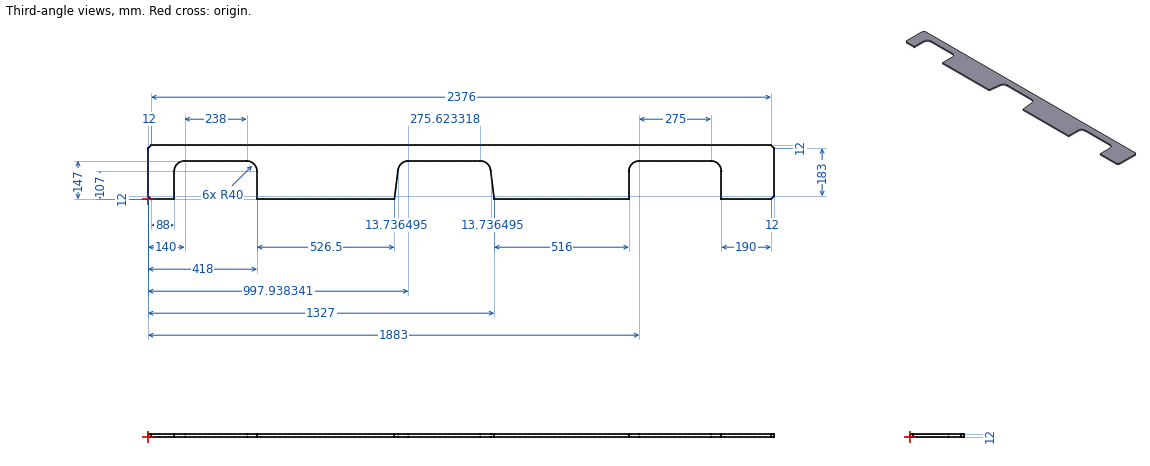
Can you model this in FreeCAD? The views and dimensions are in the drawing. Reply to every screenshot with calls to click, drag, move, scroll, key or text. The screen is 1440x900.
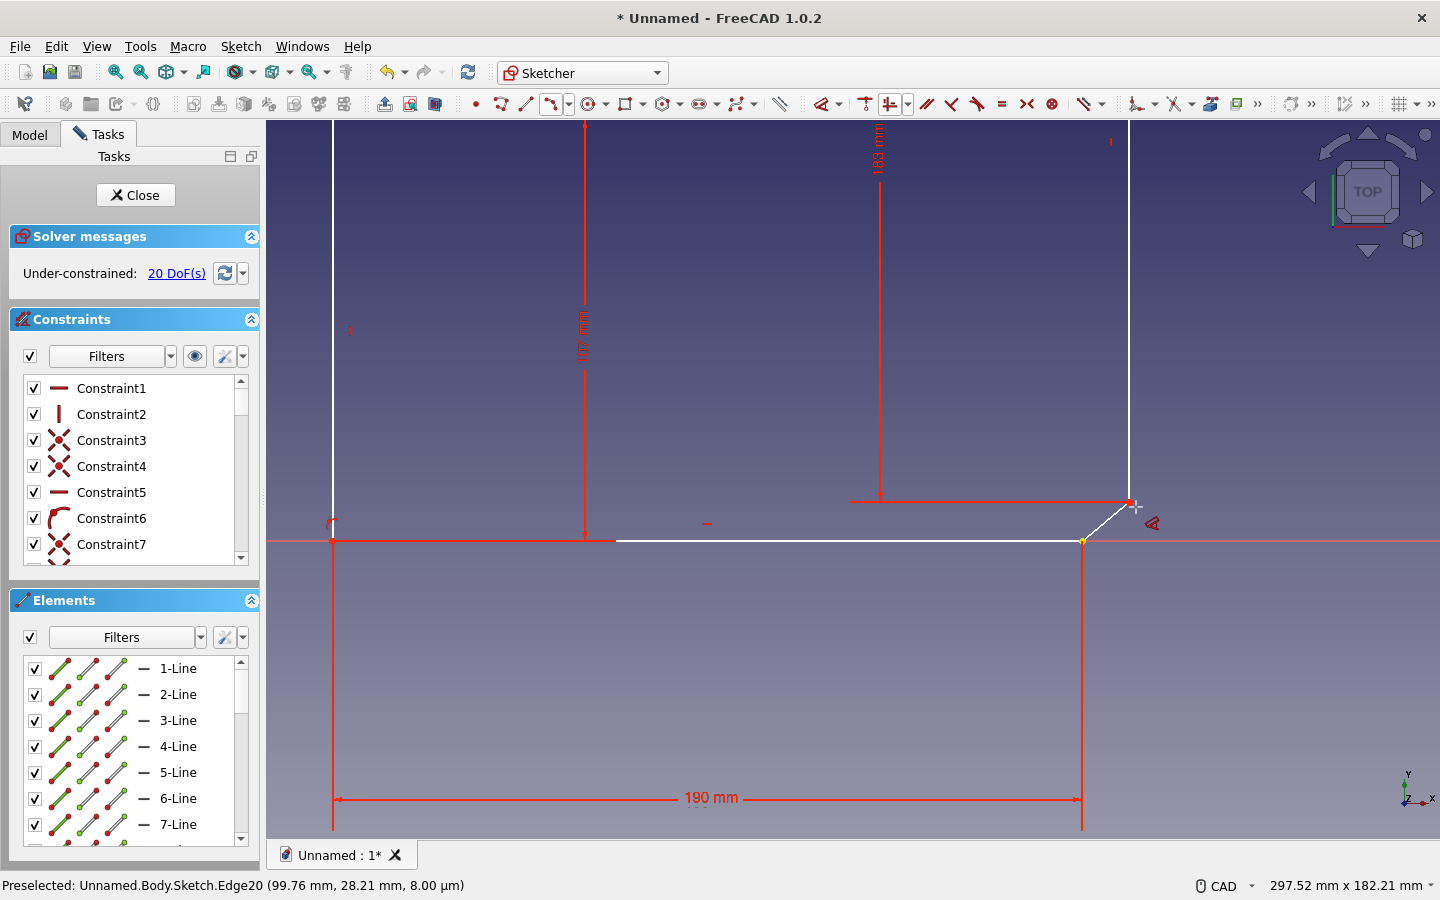
click(1129, 502)
click(1163, 522)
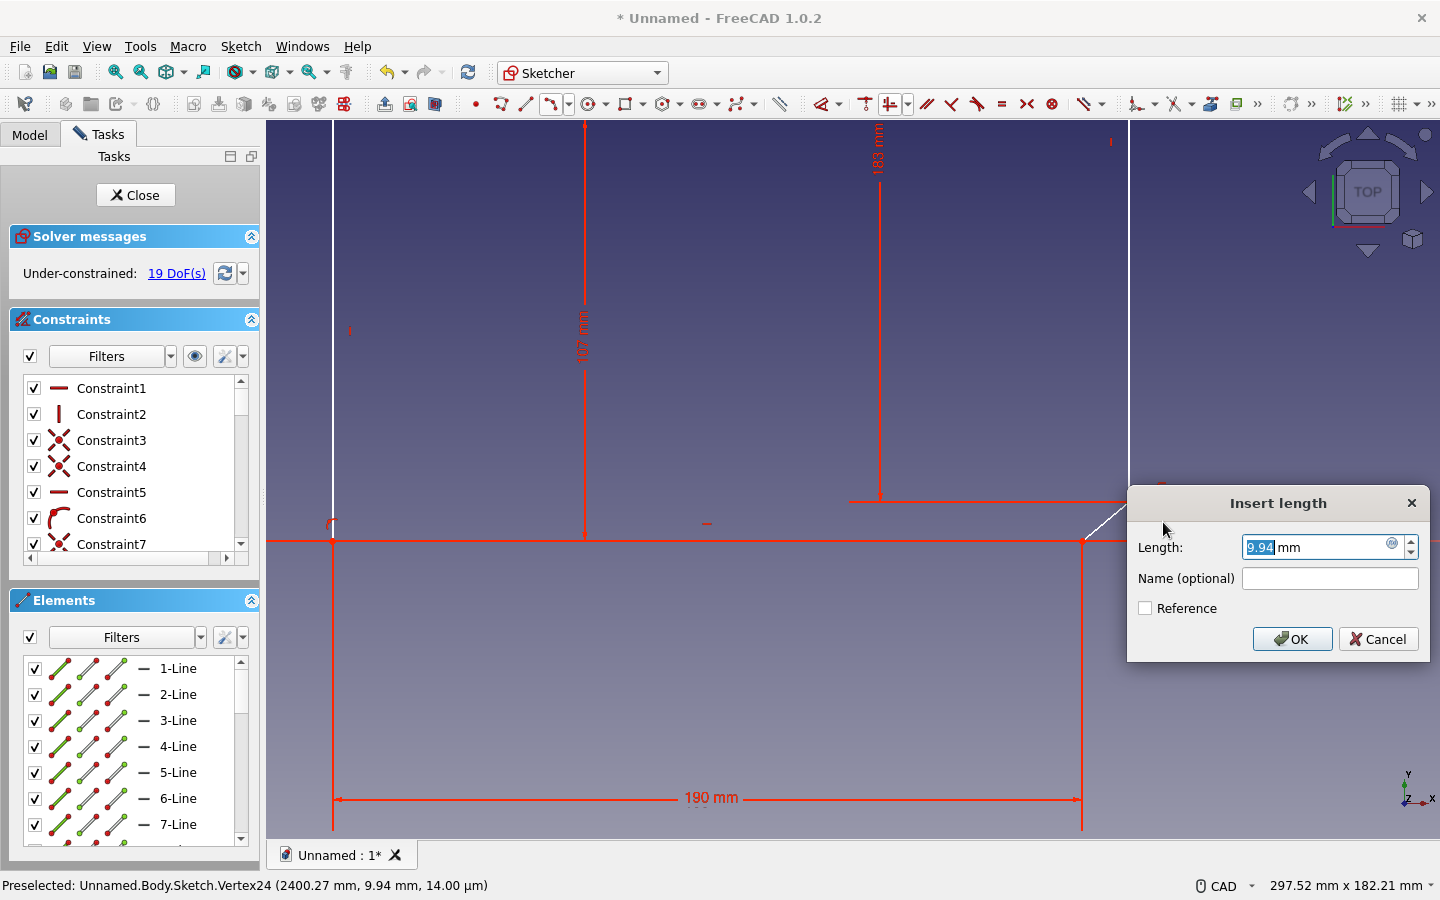
text(12)
key(Return)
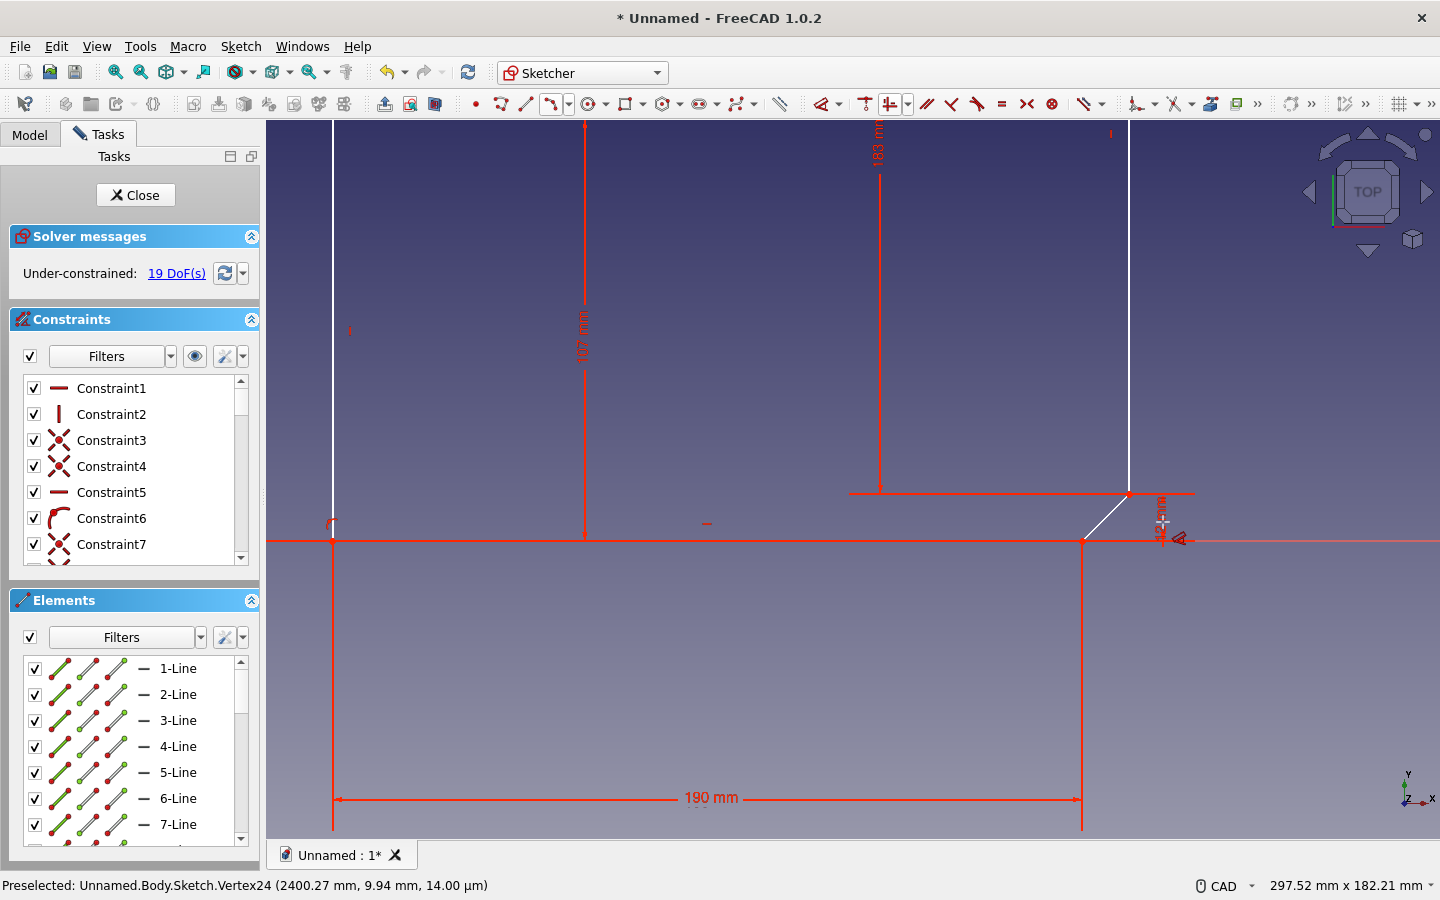
scroll(1137, 507, down, 13)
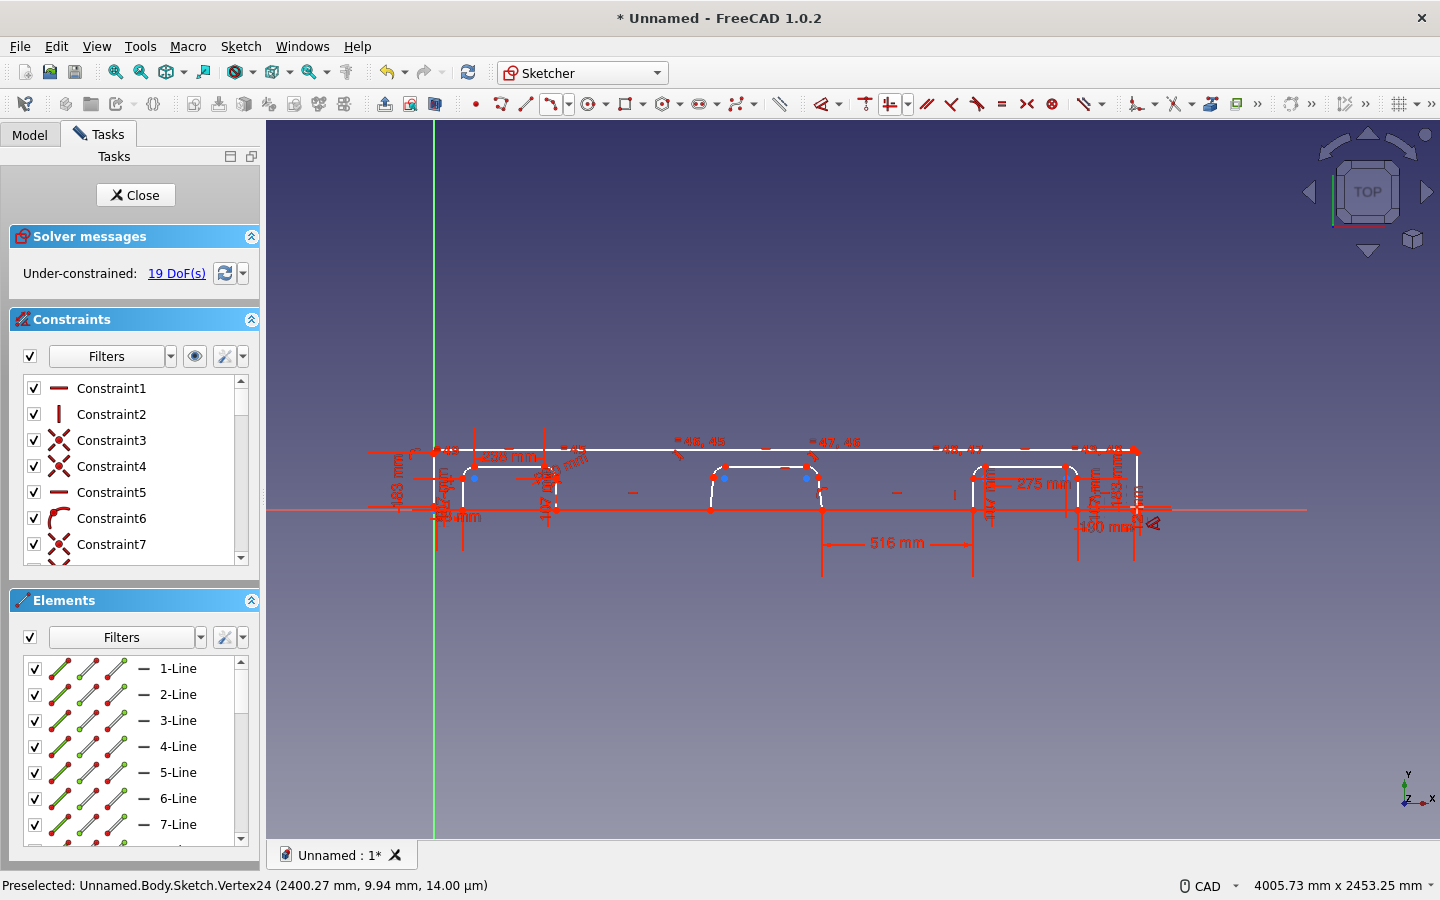
scroll(437, 450, up, 13)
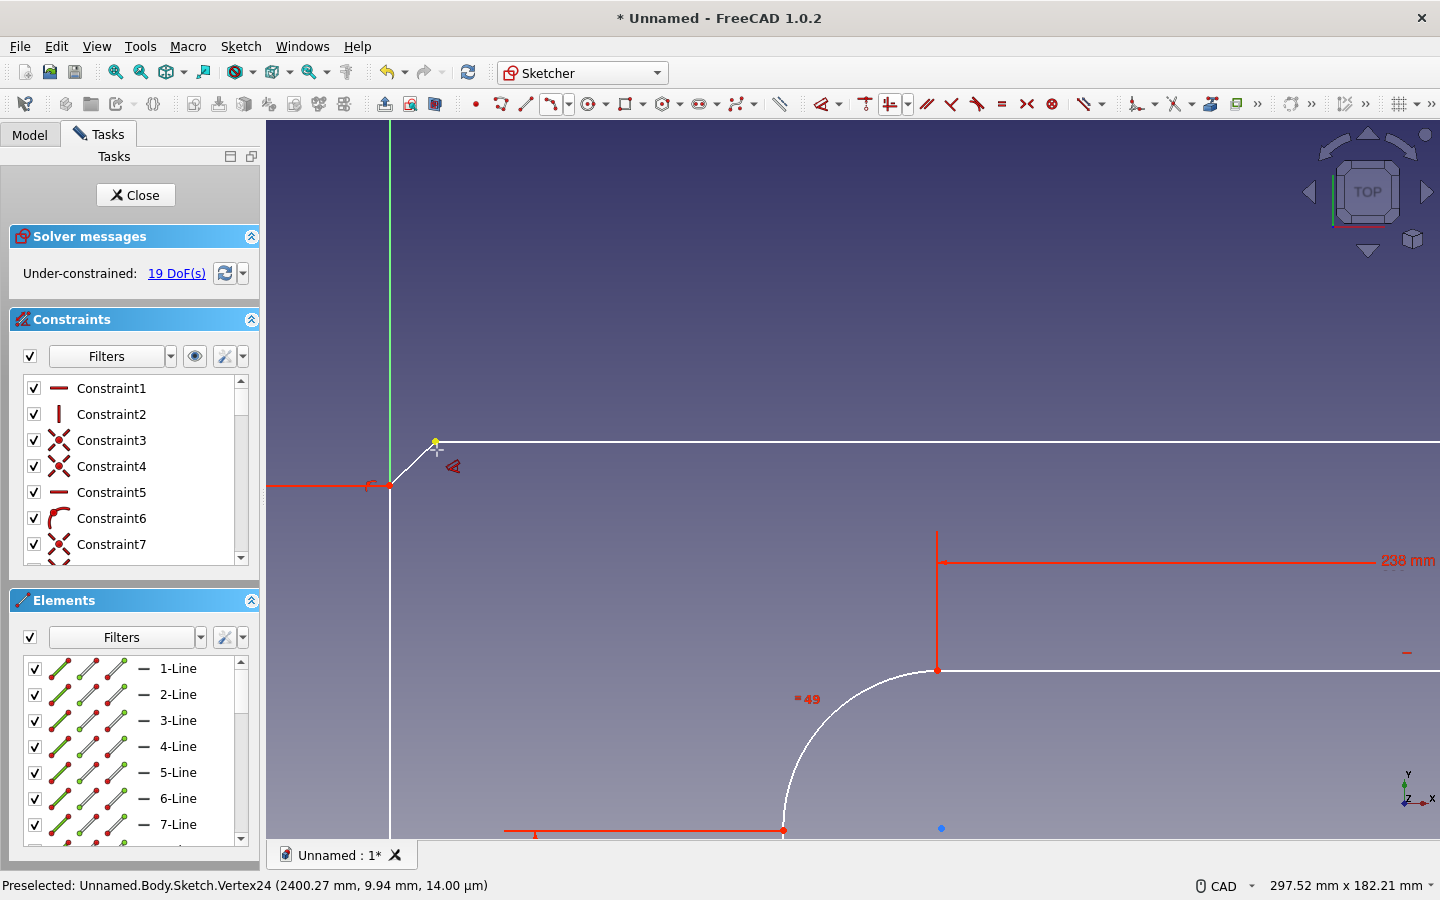
click(436, 442)
click(413, 408)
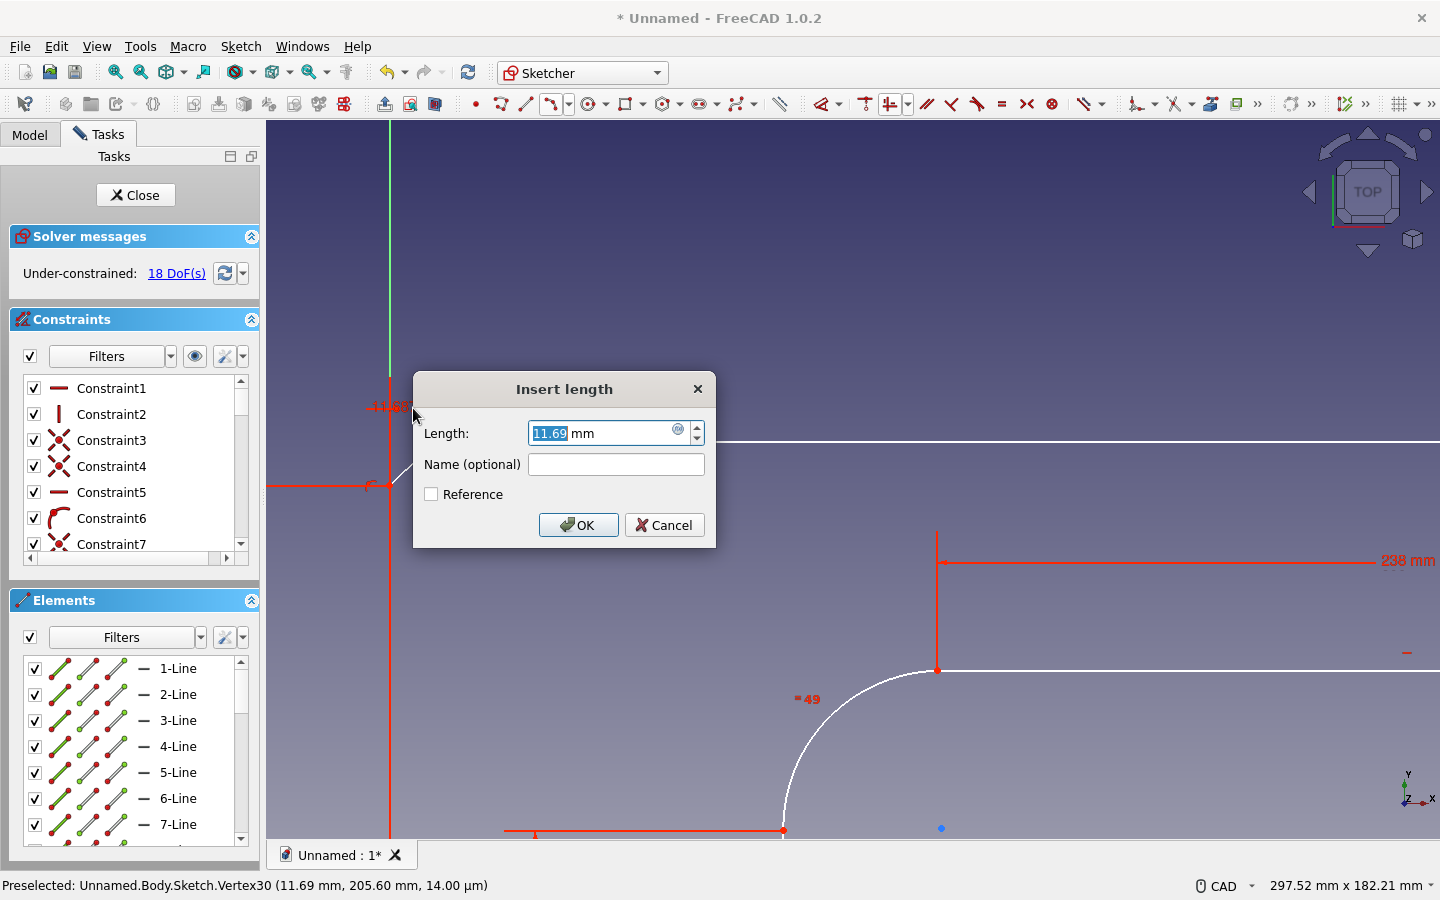
text(12)
key(Return)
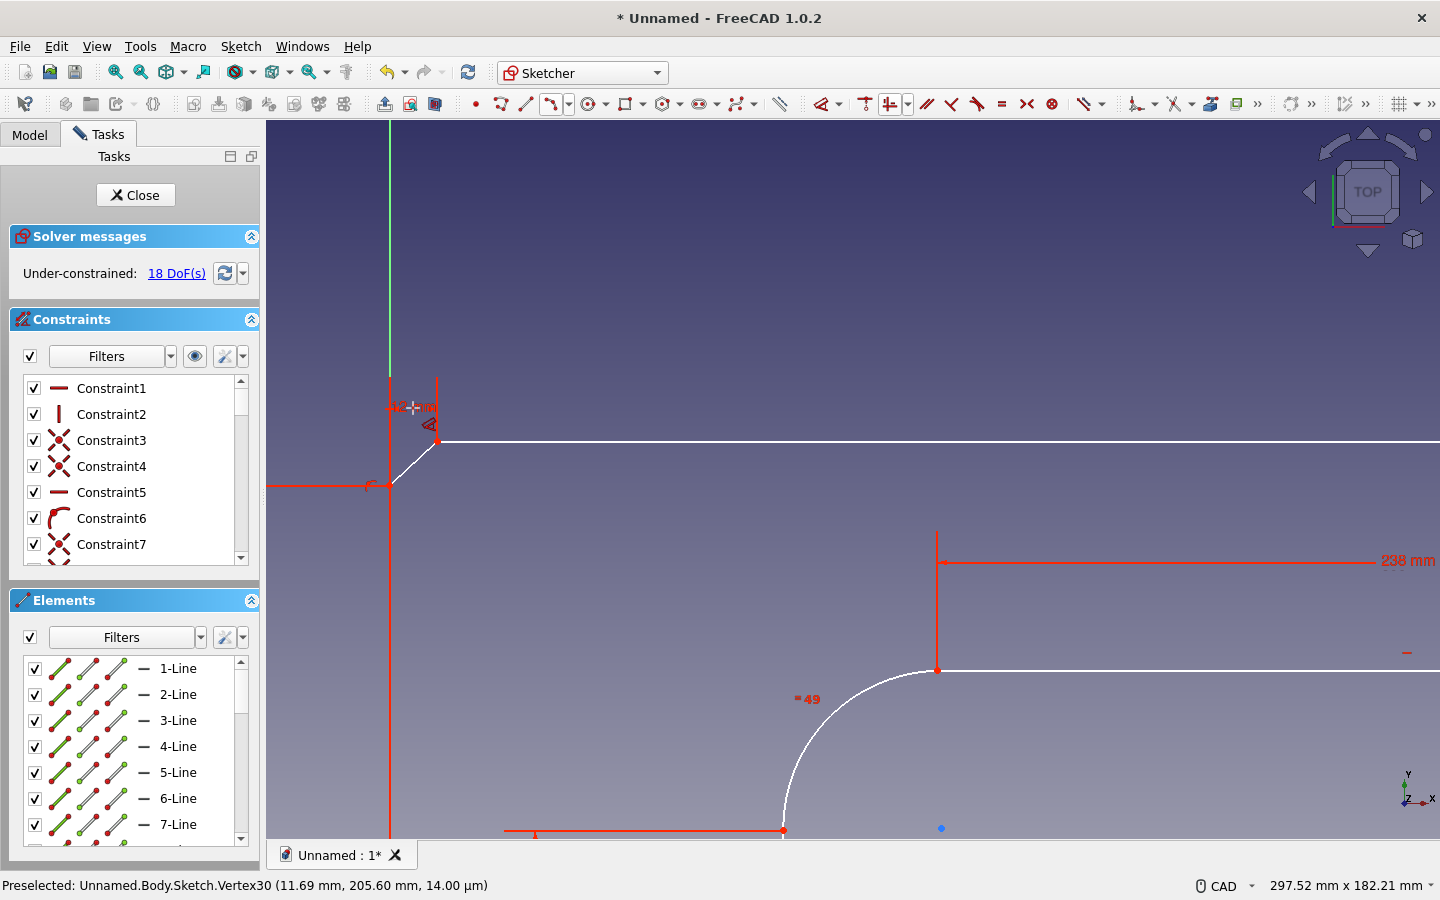
scroll(436, 450, down, 13)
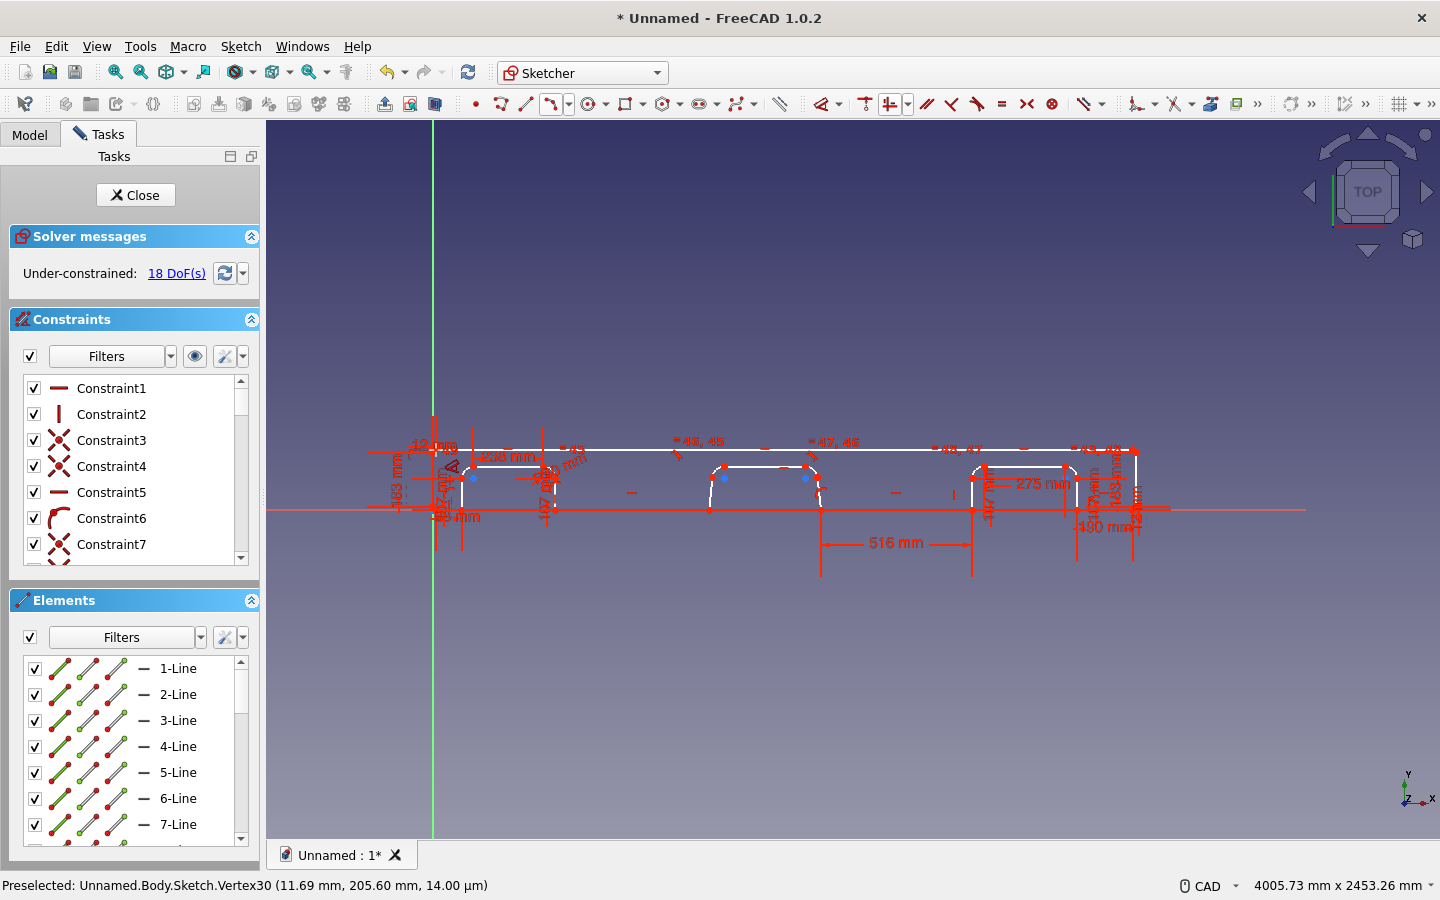
scroll(433, 507, up, 13)